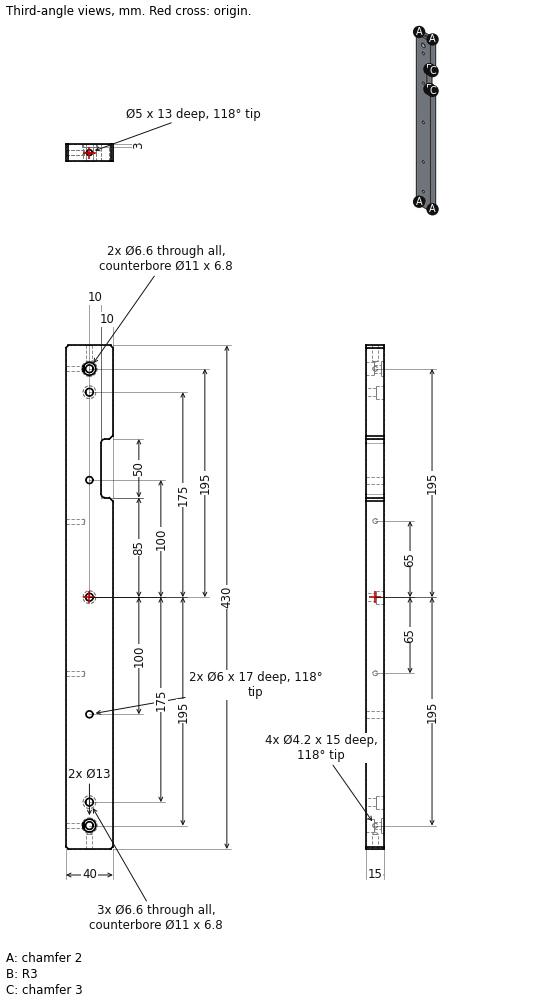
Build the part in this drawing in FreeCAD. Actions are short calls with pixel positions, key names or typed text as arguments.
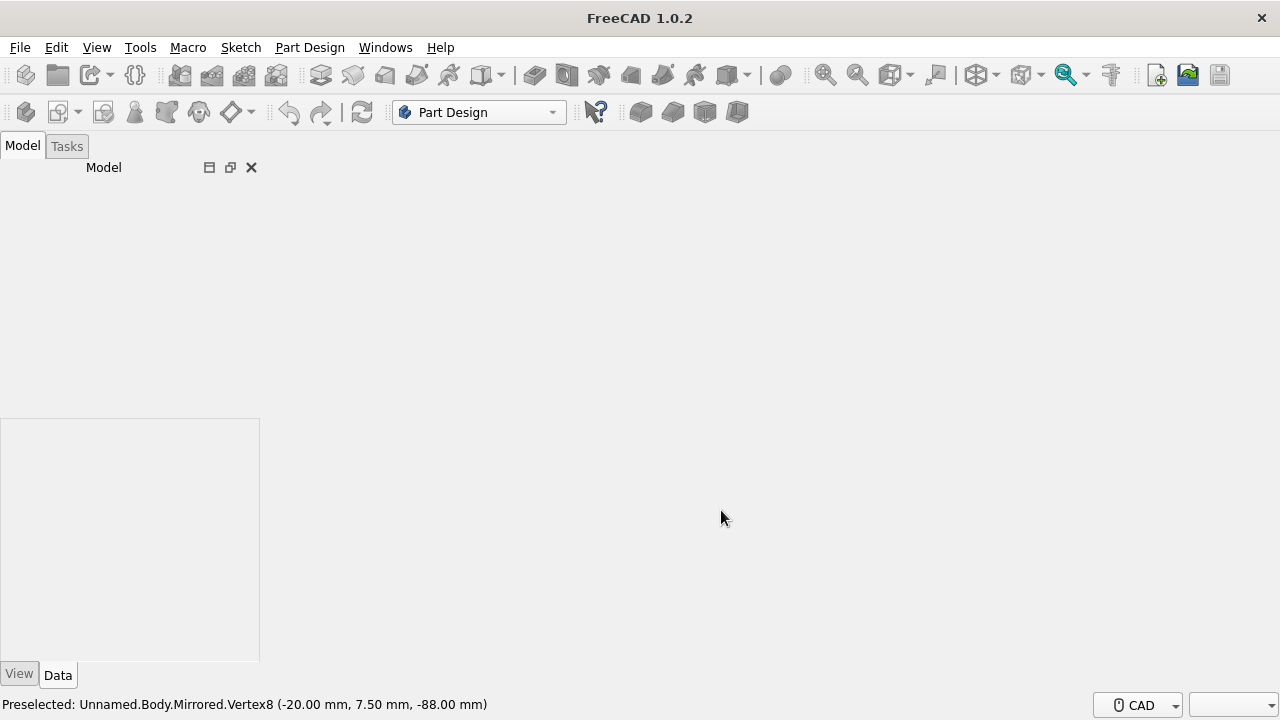
click(1156, 76)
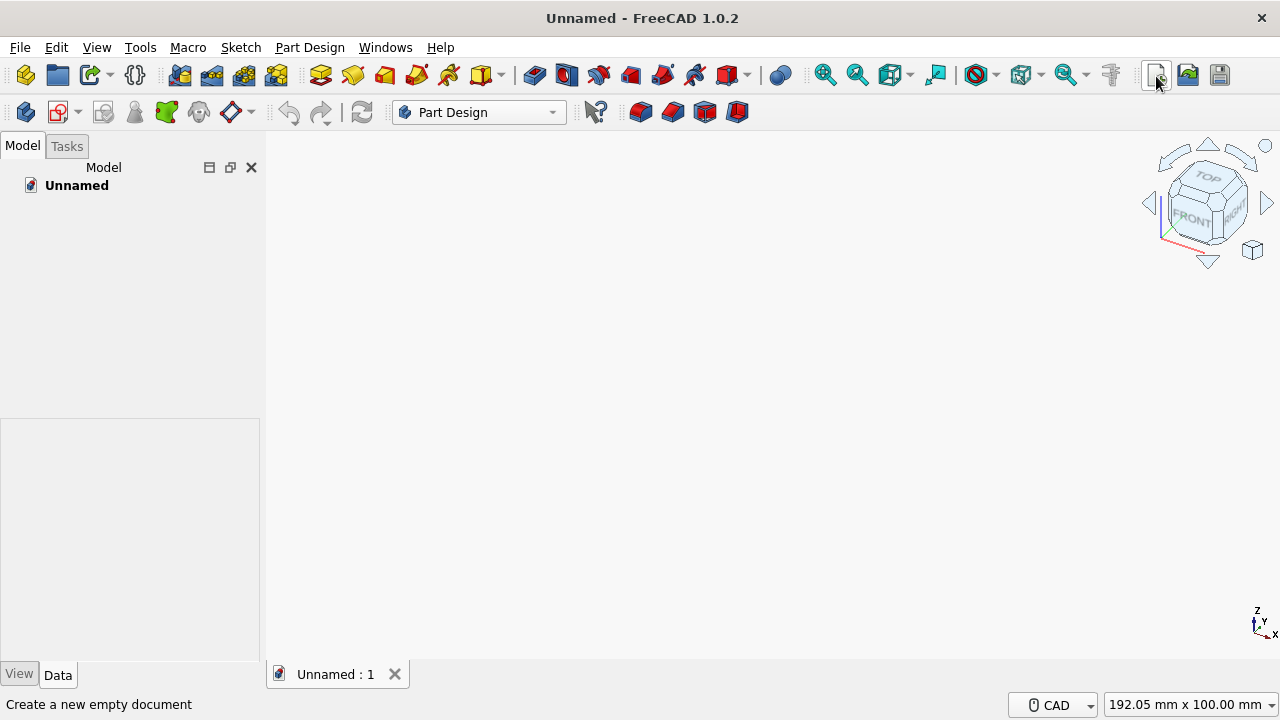
click(58, 112)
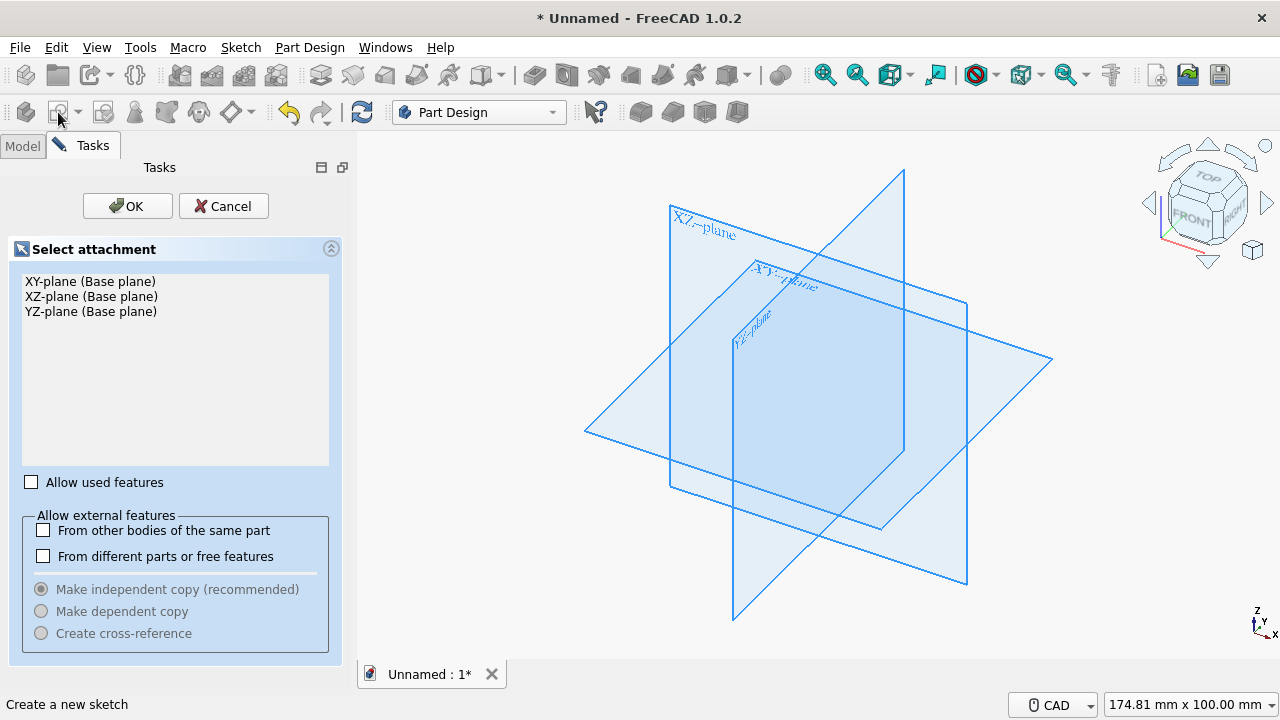
click(82, 296)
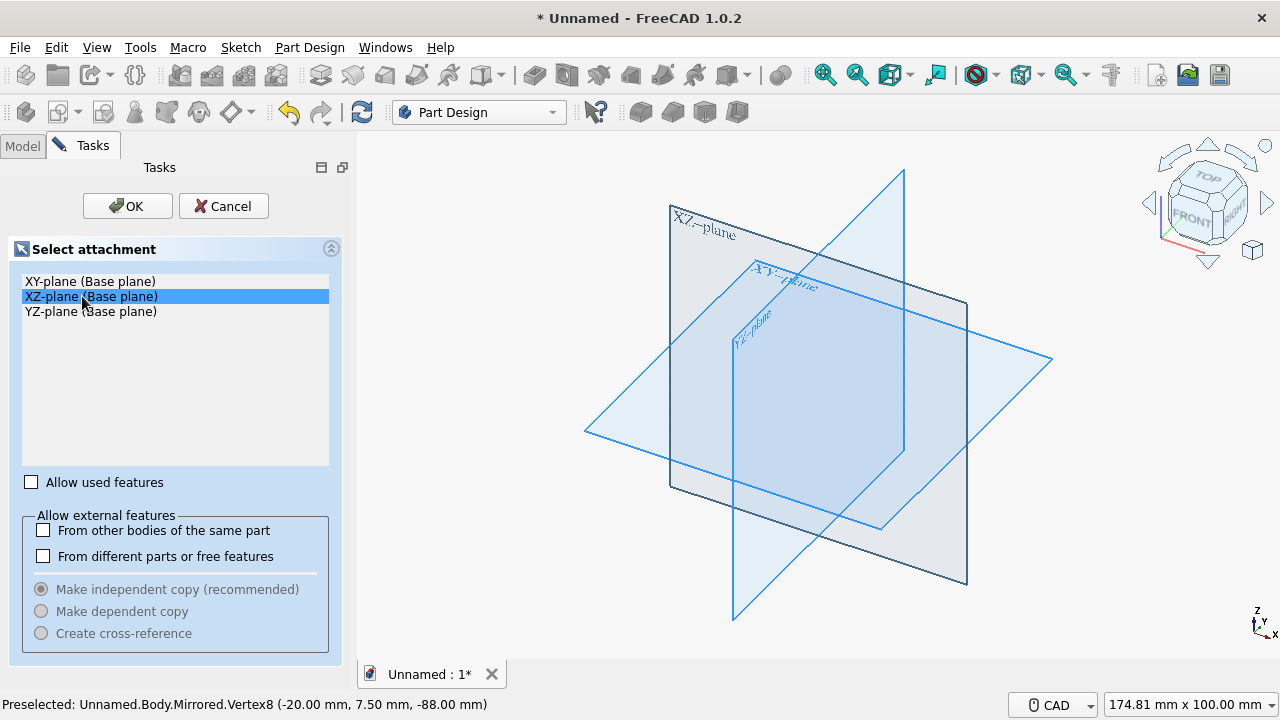
click(128, 206)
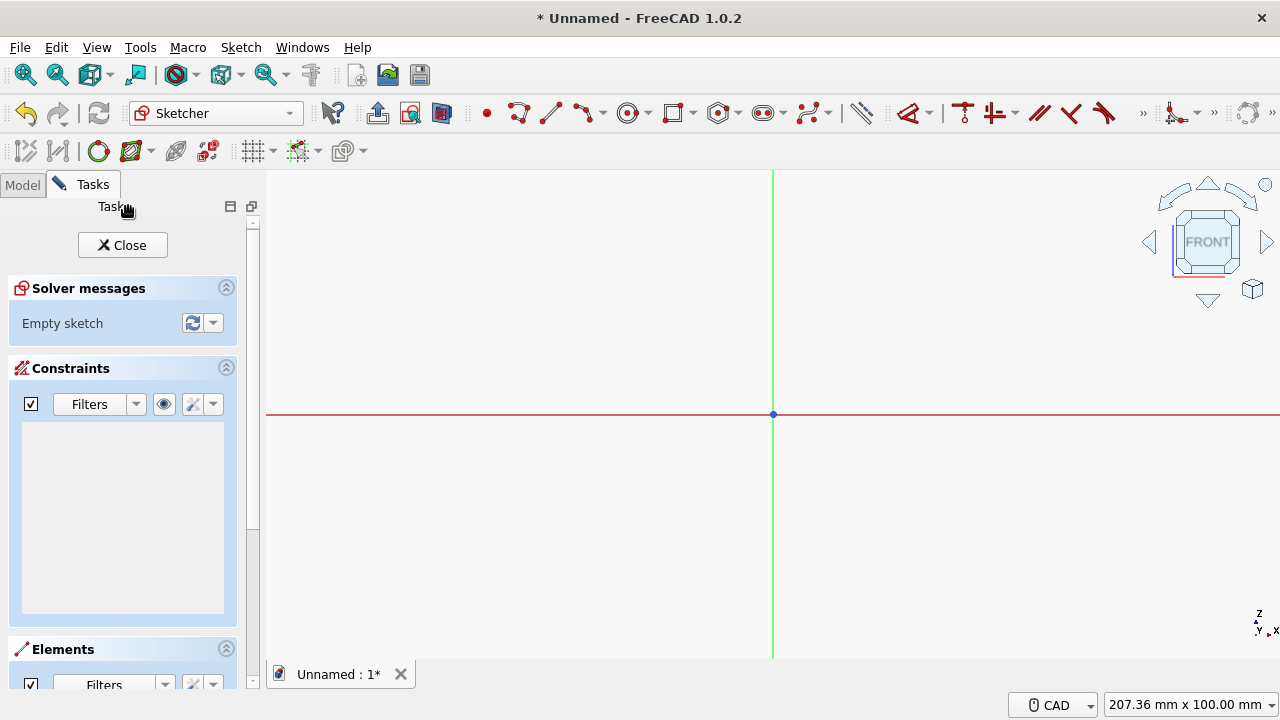
scroll(694, 414, down, 10)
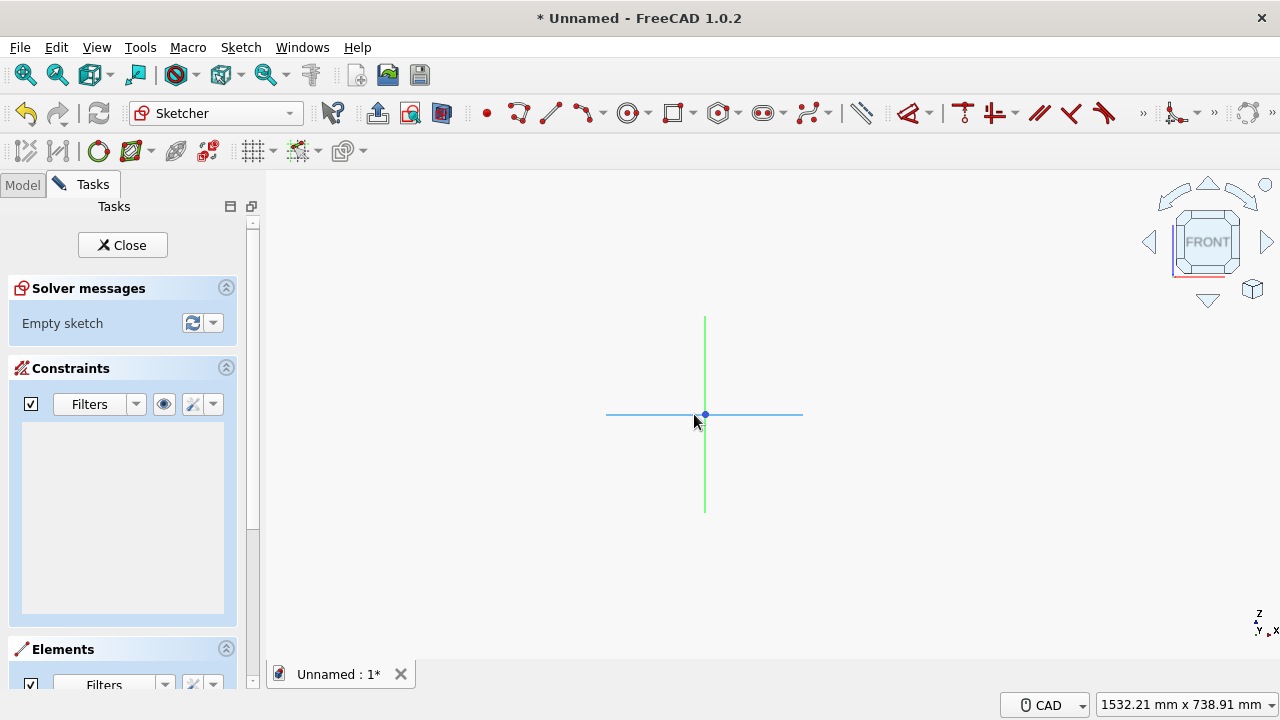
key(g)
key(v)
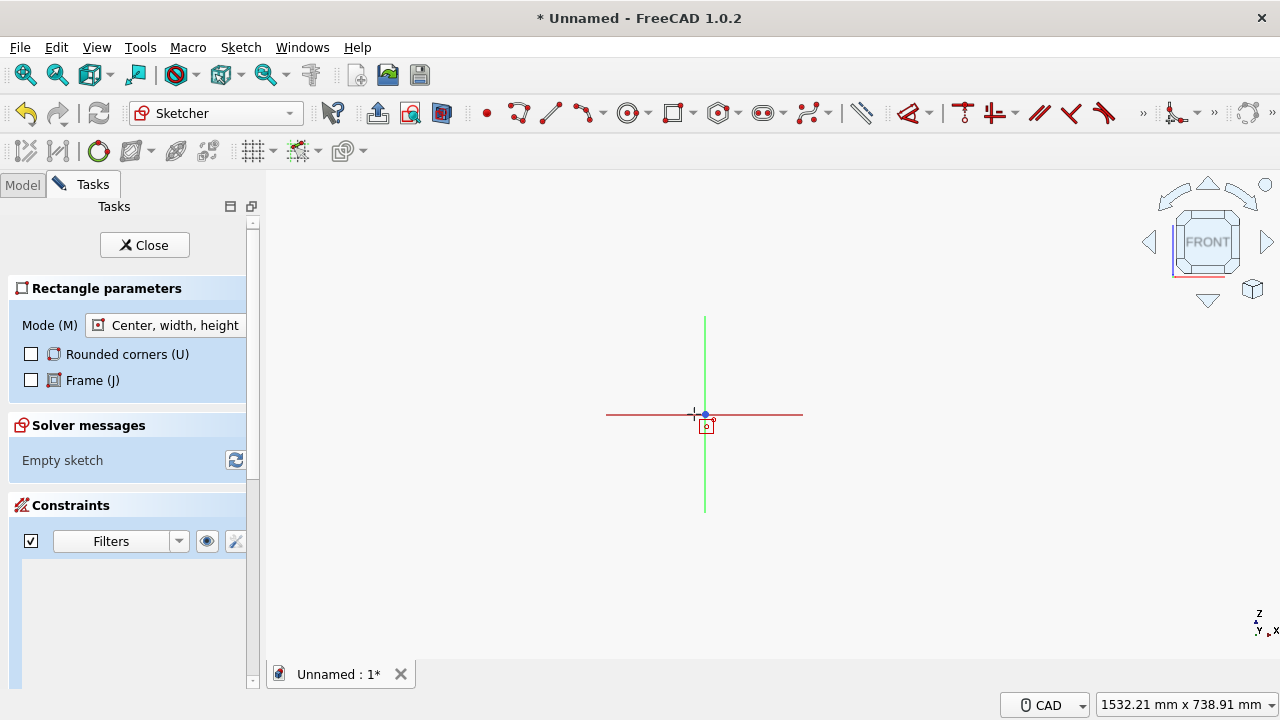
click(705, 414)
move(718, 272)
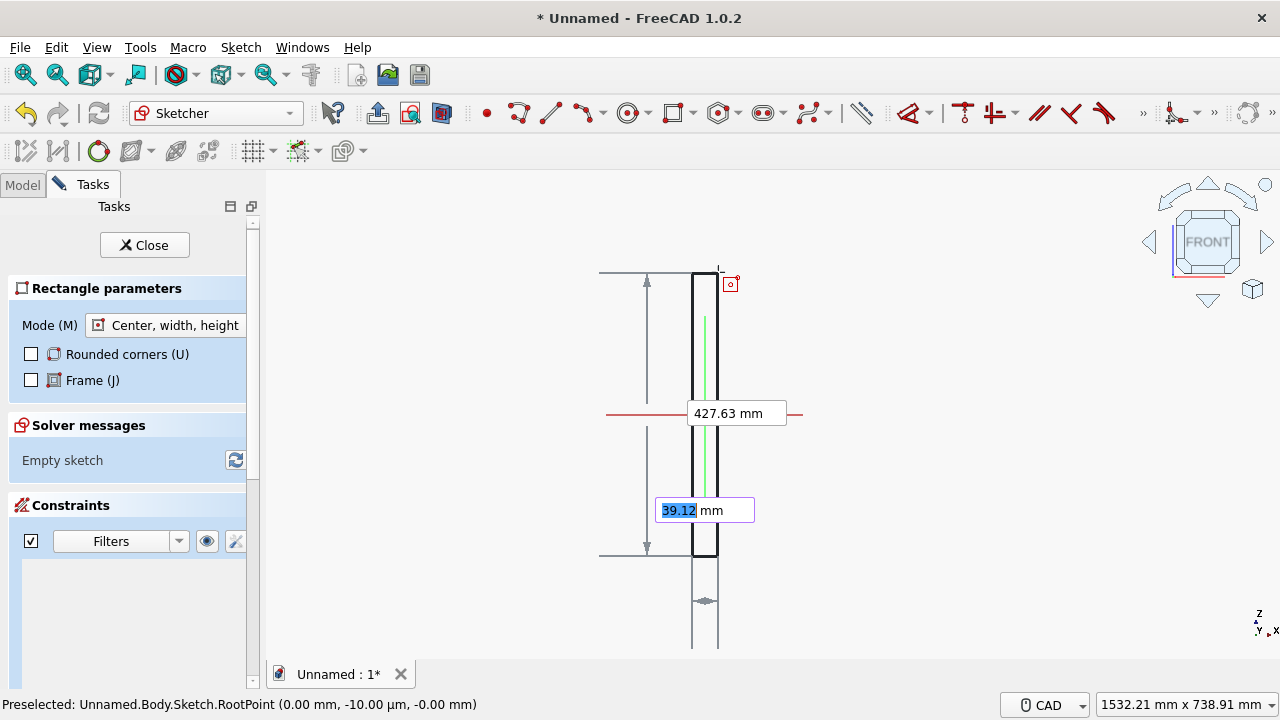
text(40)
key(Tab)
text(430)
key(Return)
key(Escape)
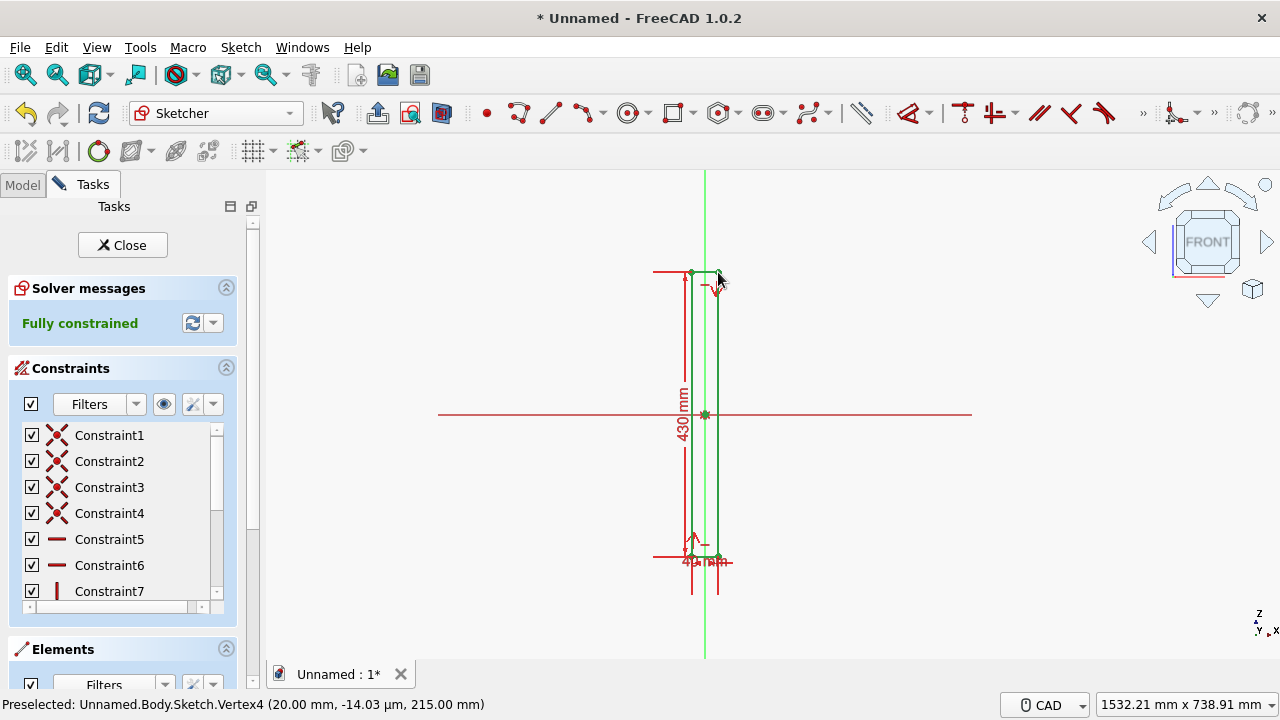
click(123, 245)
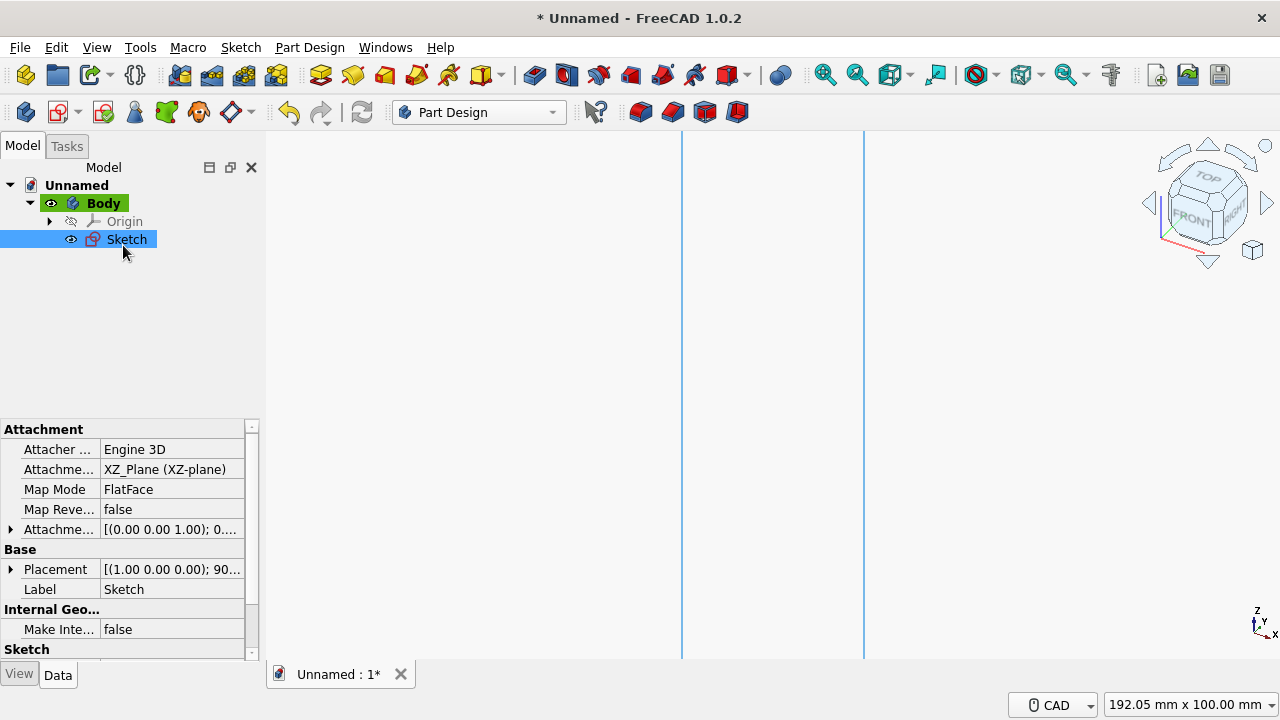
click(322, 76)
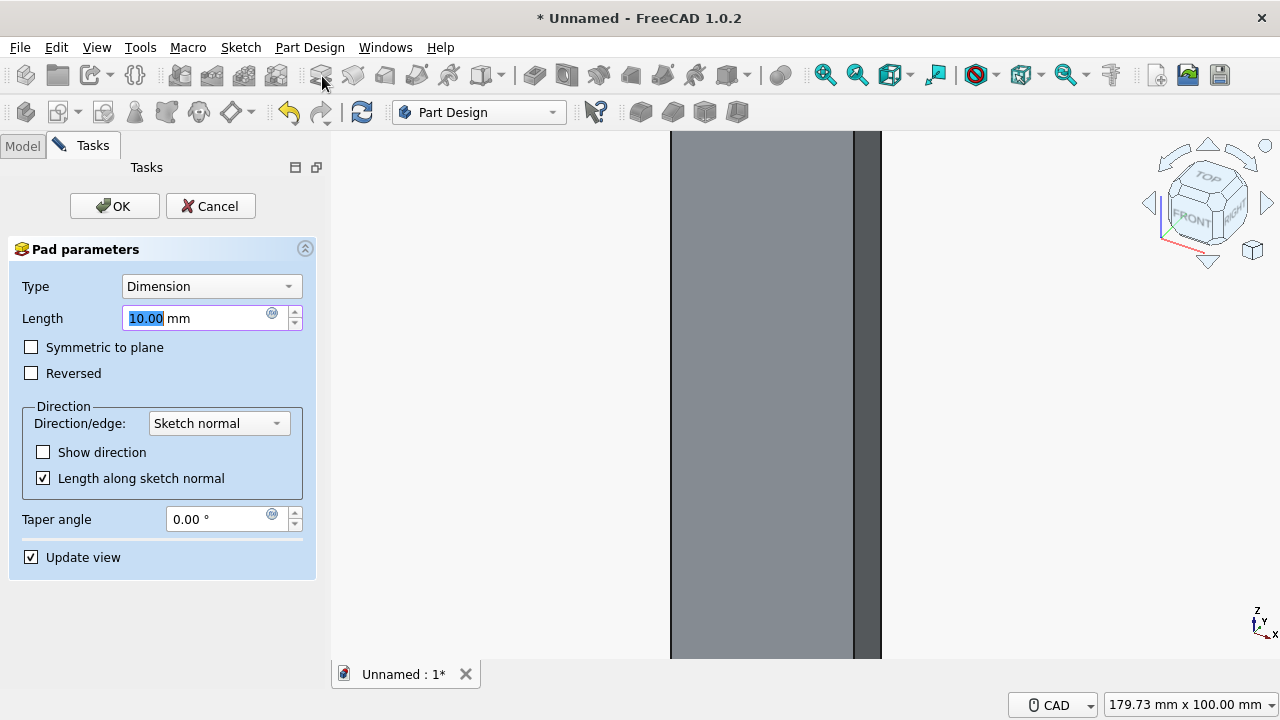
text(15)
key(Tab)